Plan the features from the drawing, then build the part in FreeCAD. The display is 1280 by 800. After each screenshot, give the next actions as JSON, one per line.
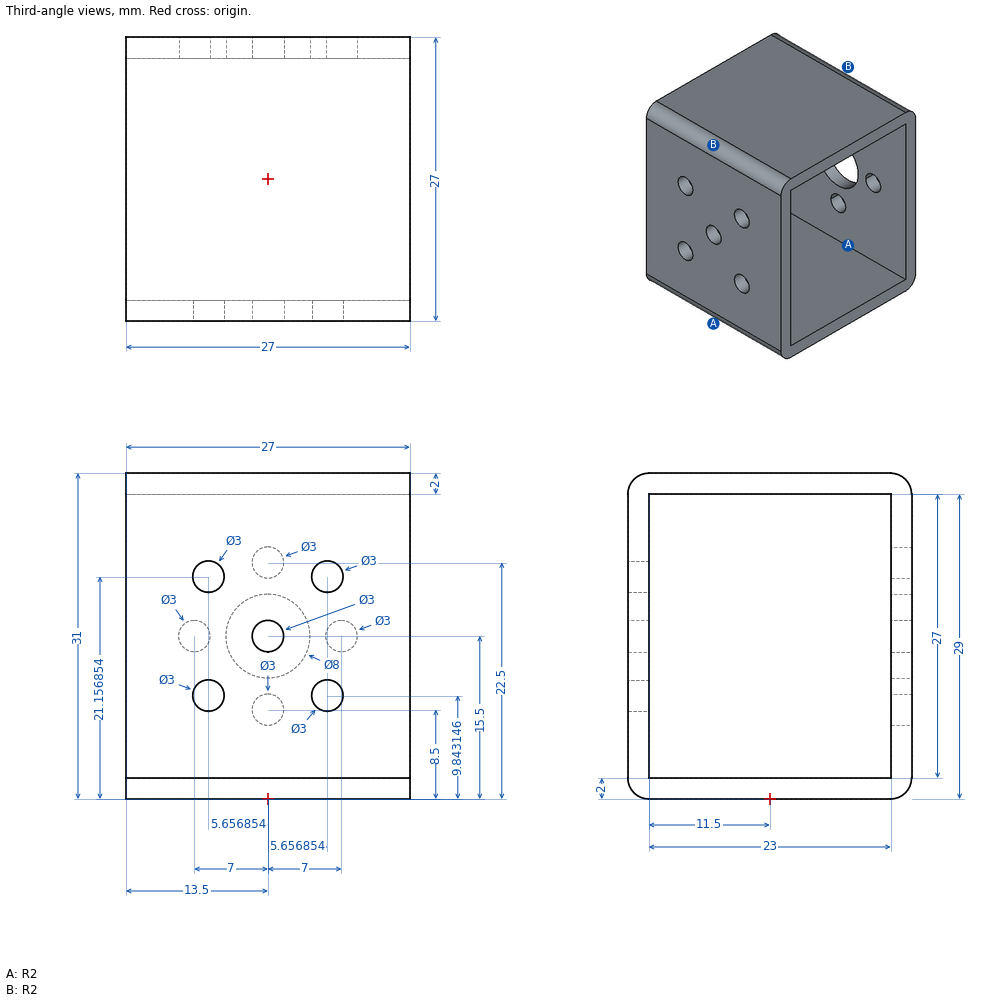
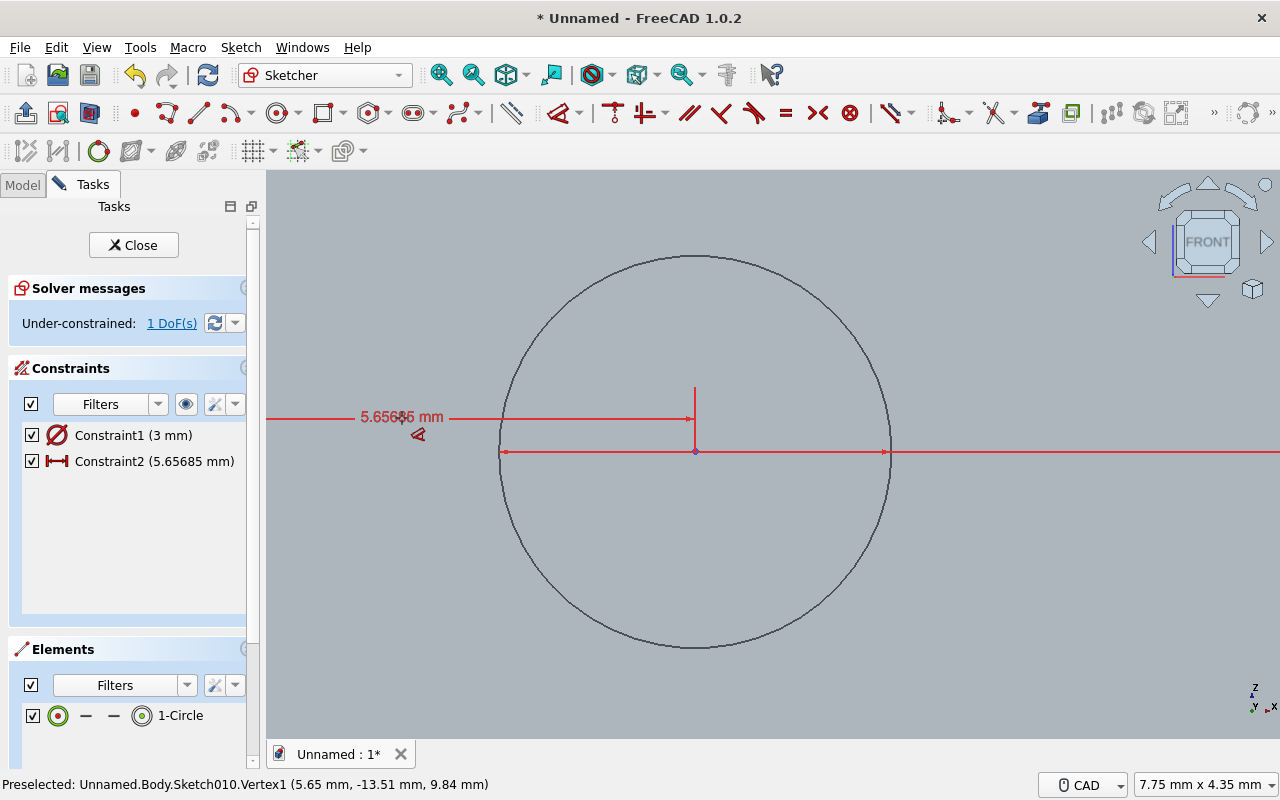
{"action": "left_click", "coordinate": [695, 452]}
{"action": "left_click", "coordinate": [729, 581]}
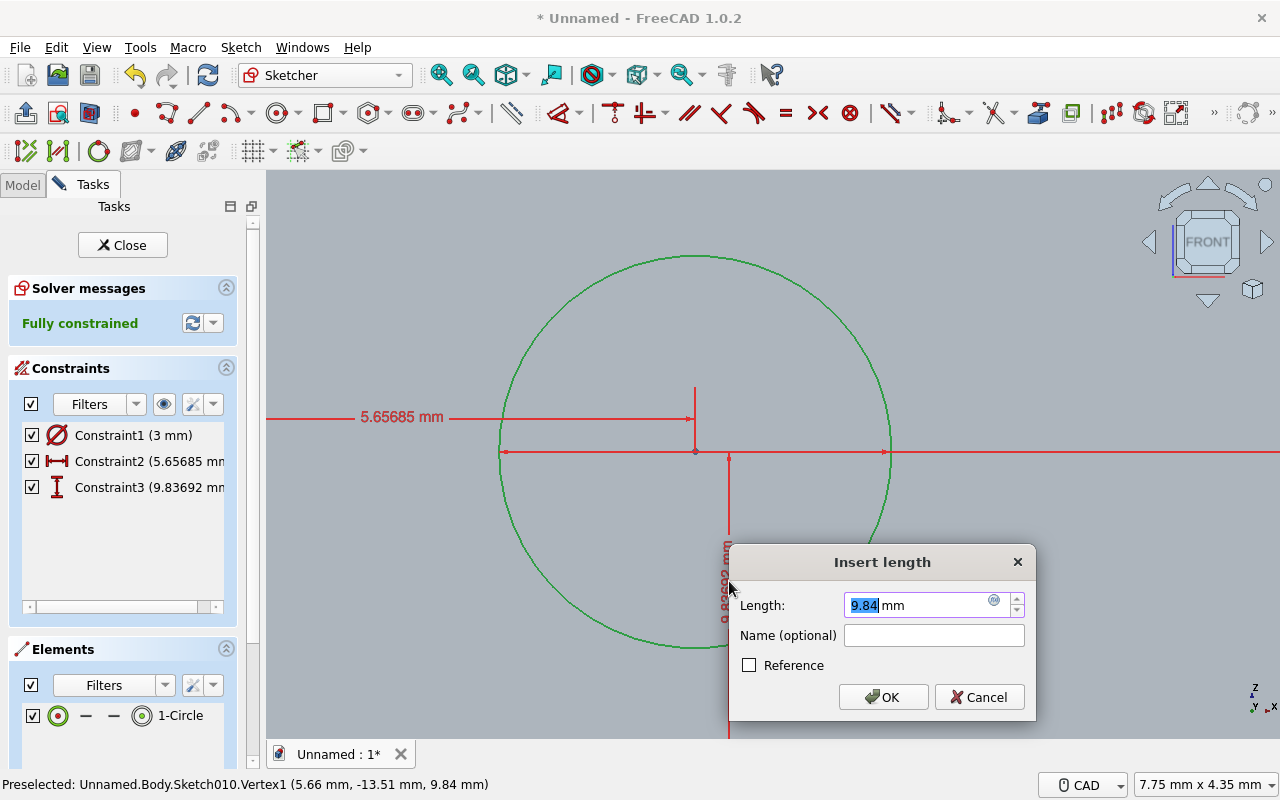
{"action": "type", "text": "9.843146"}
{"action": "key", "text": "Return"}
{"action": "key", "text": "Escape"}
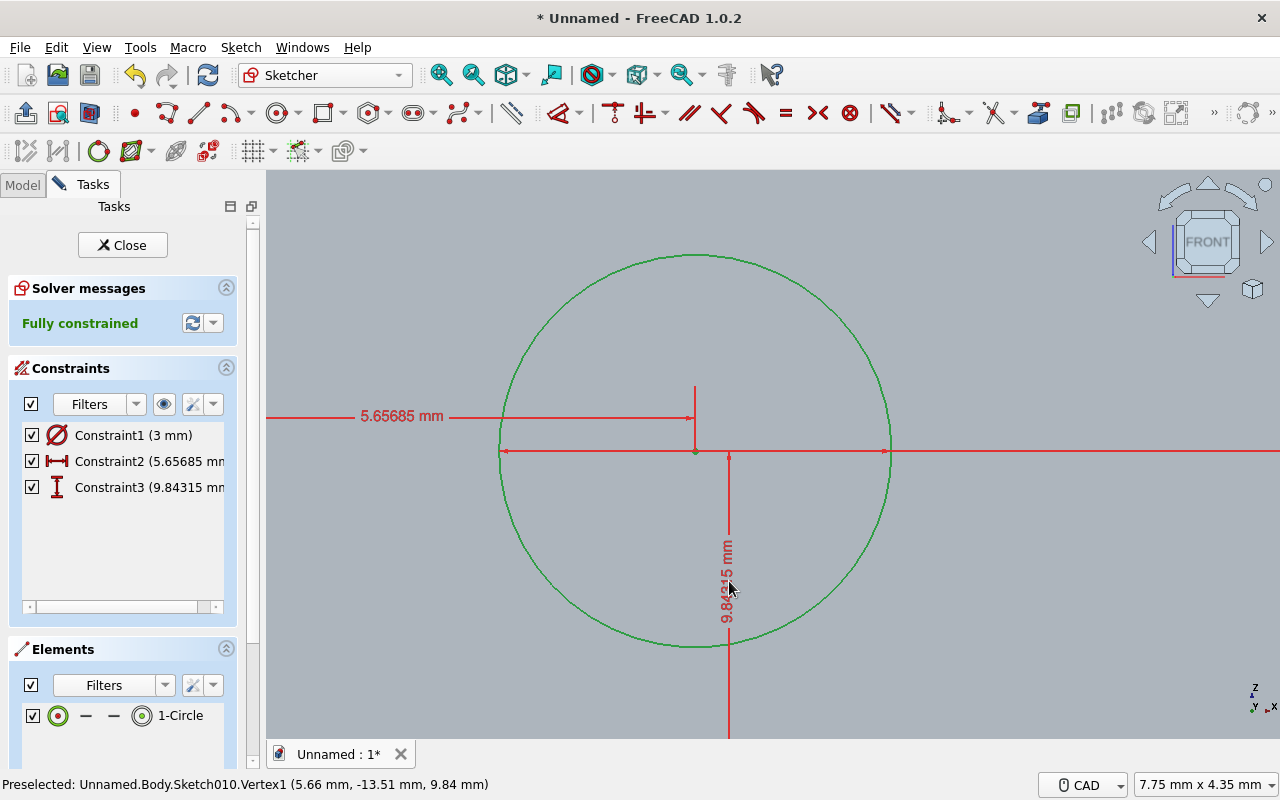
{"action": "left_click", "coordinate": [123, 245]}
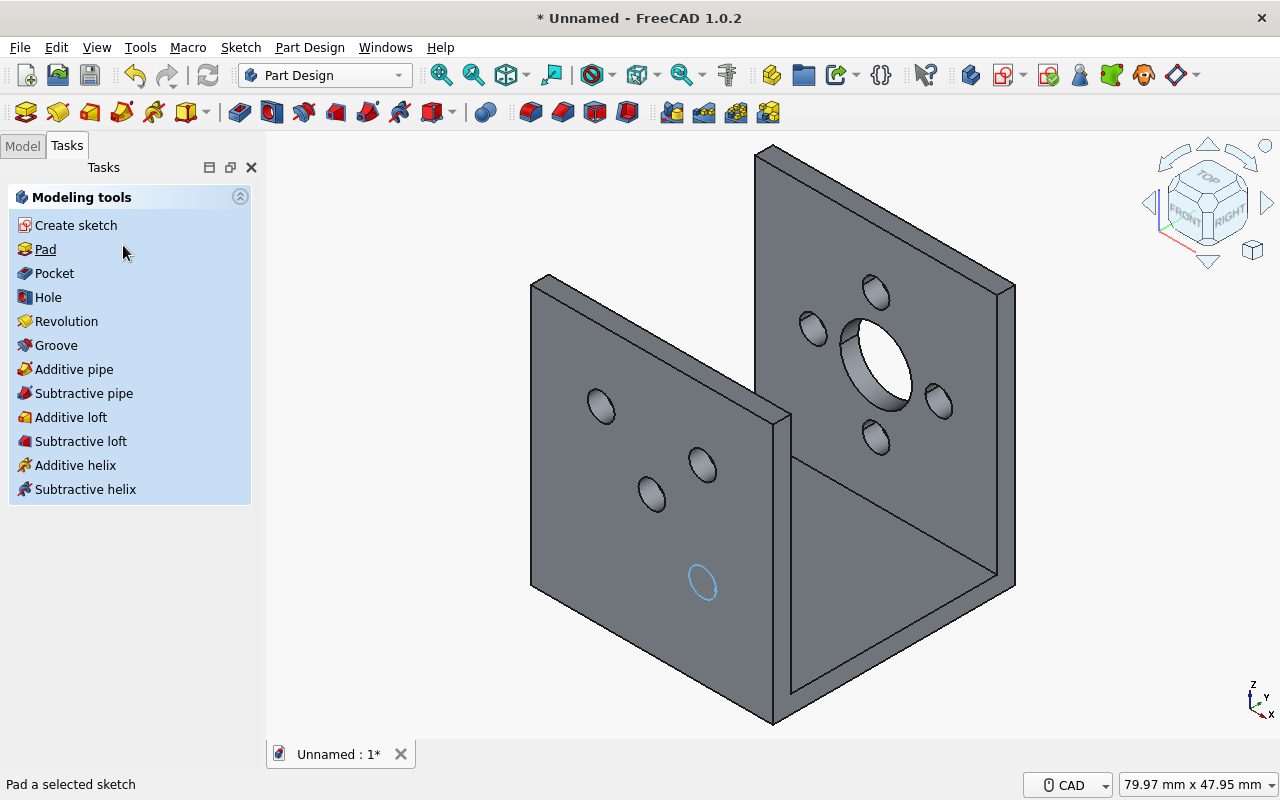
{"action": "left_click", "coordinate": [240, 112]}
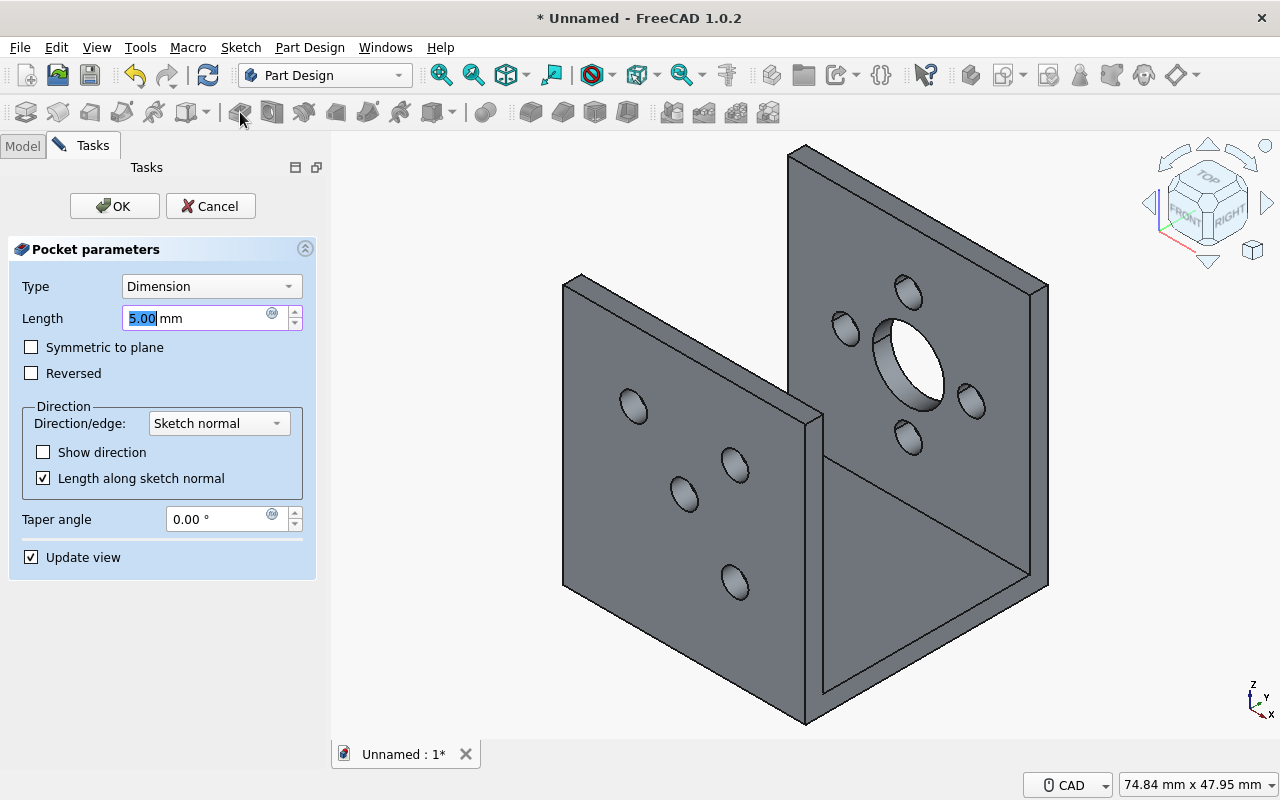
{"action": "left_click", "coordinate": [212, 286]}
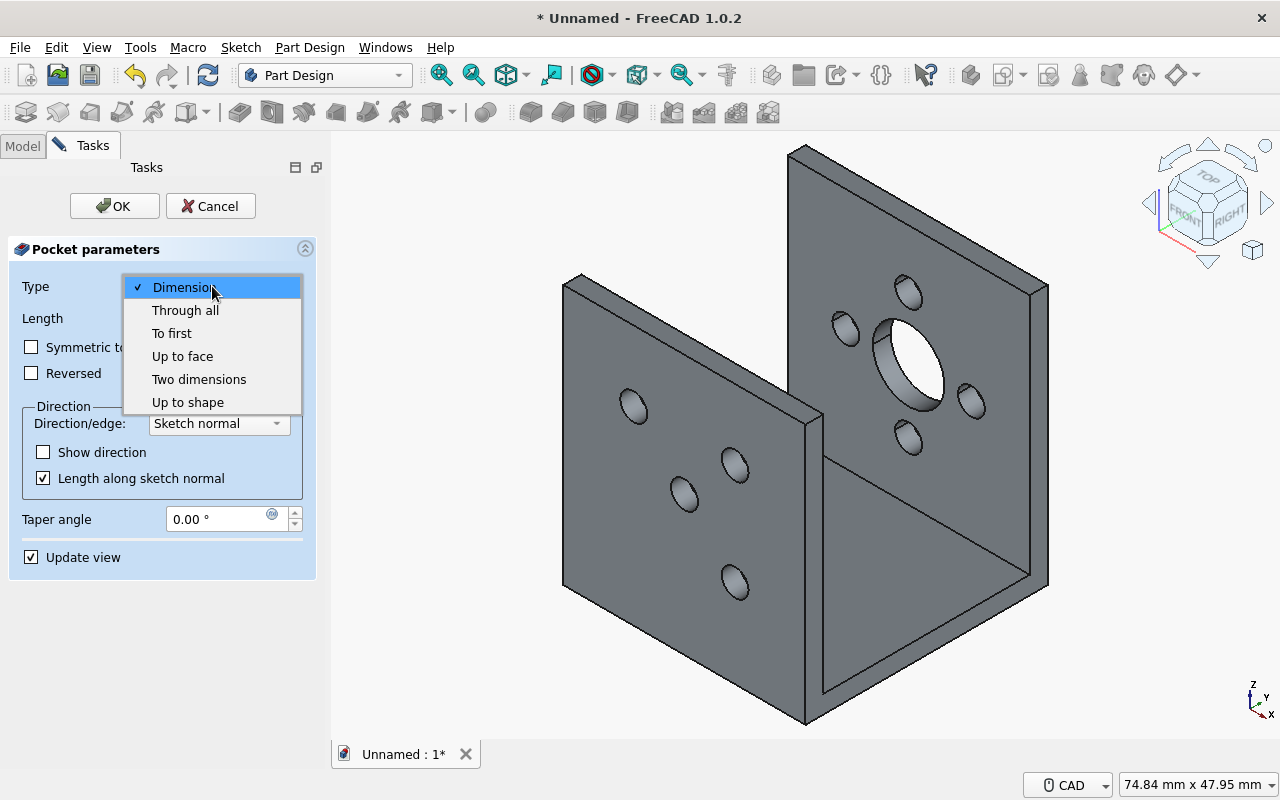
{"action": "left_click", "coordinate": [212, 334]}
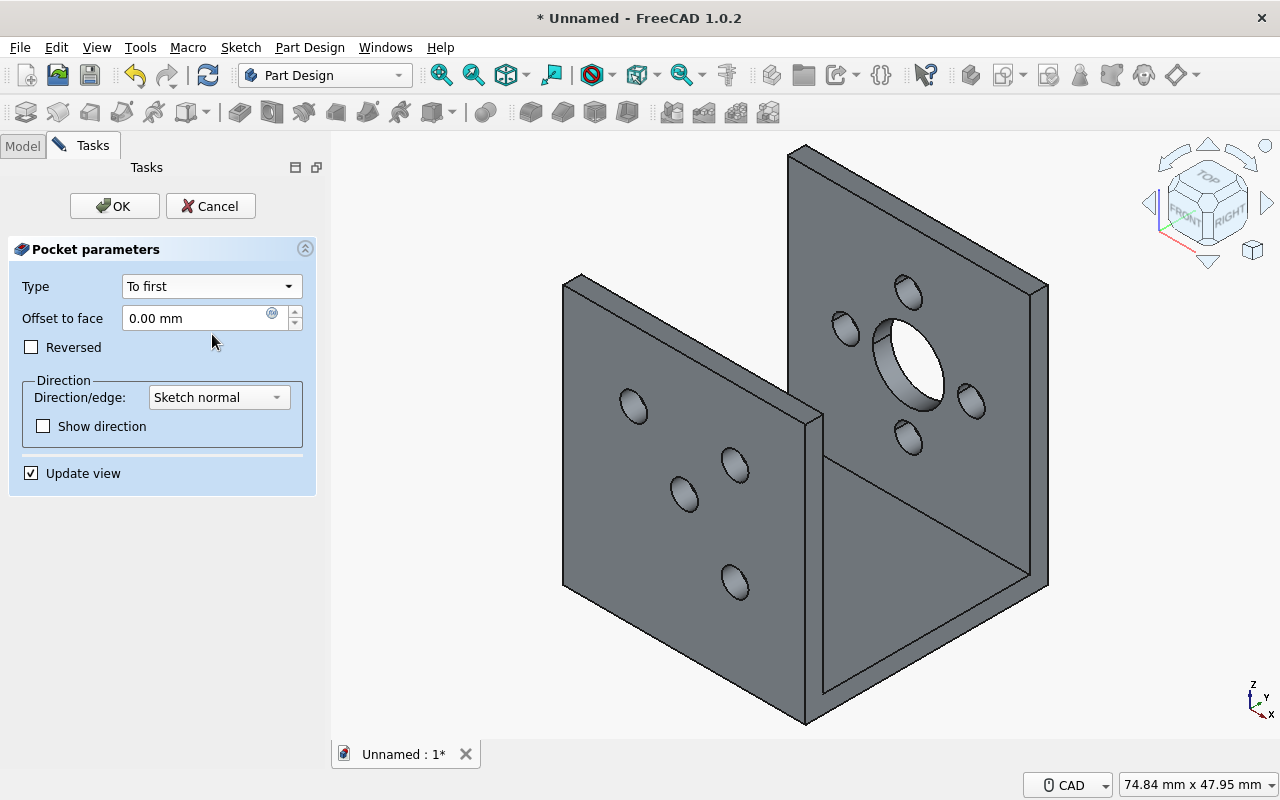
{"action": "left_click", "coordinate": [115, 206]}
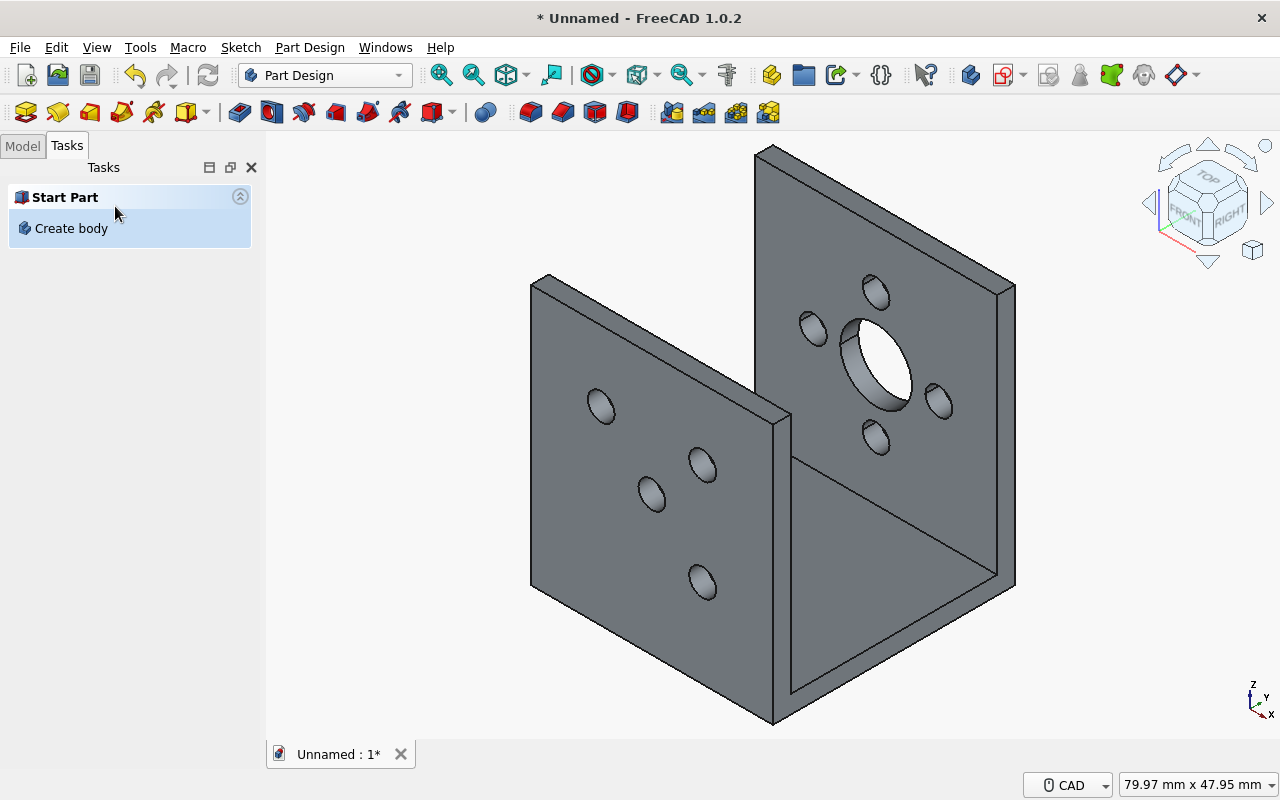
{"action": "left_click", "coordinate": [617, 570]}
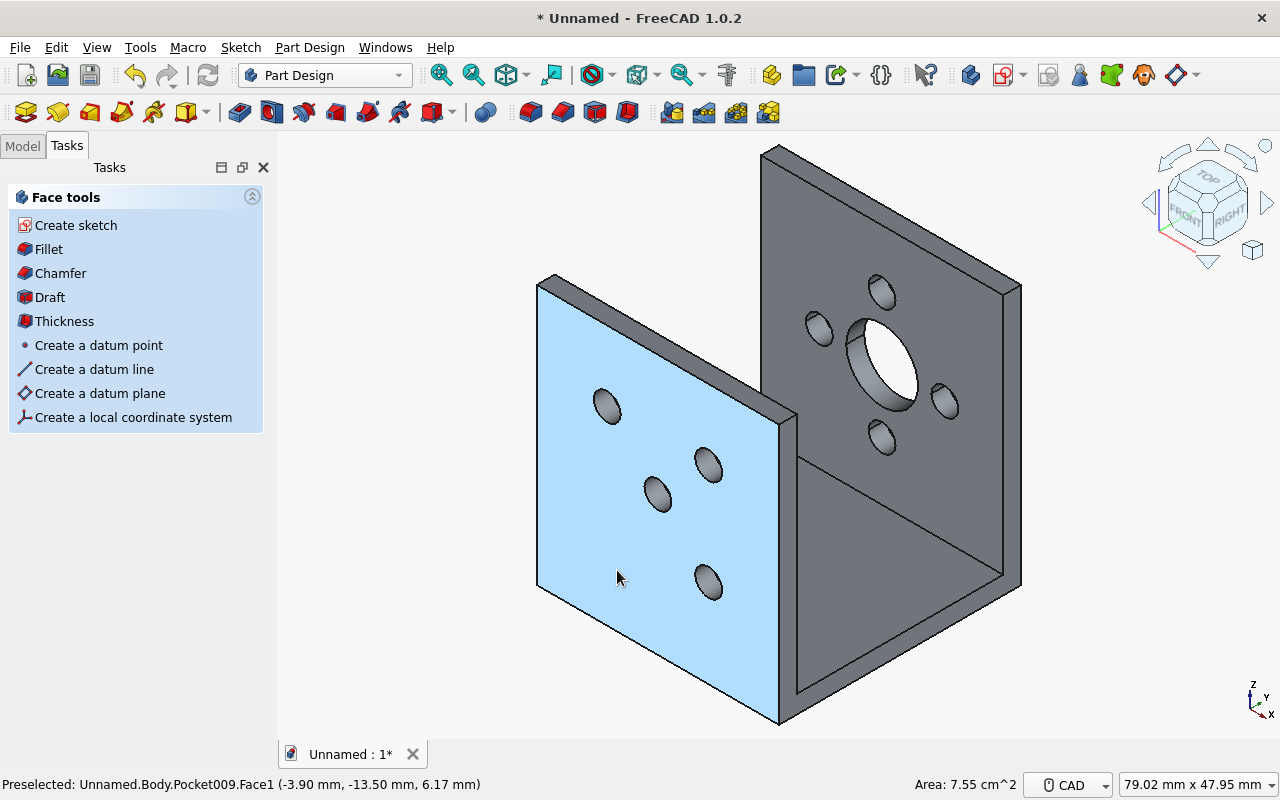
{"action": "left_click", "coordinate": [1004, 76]}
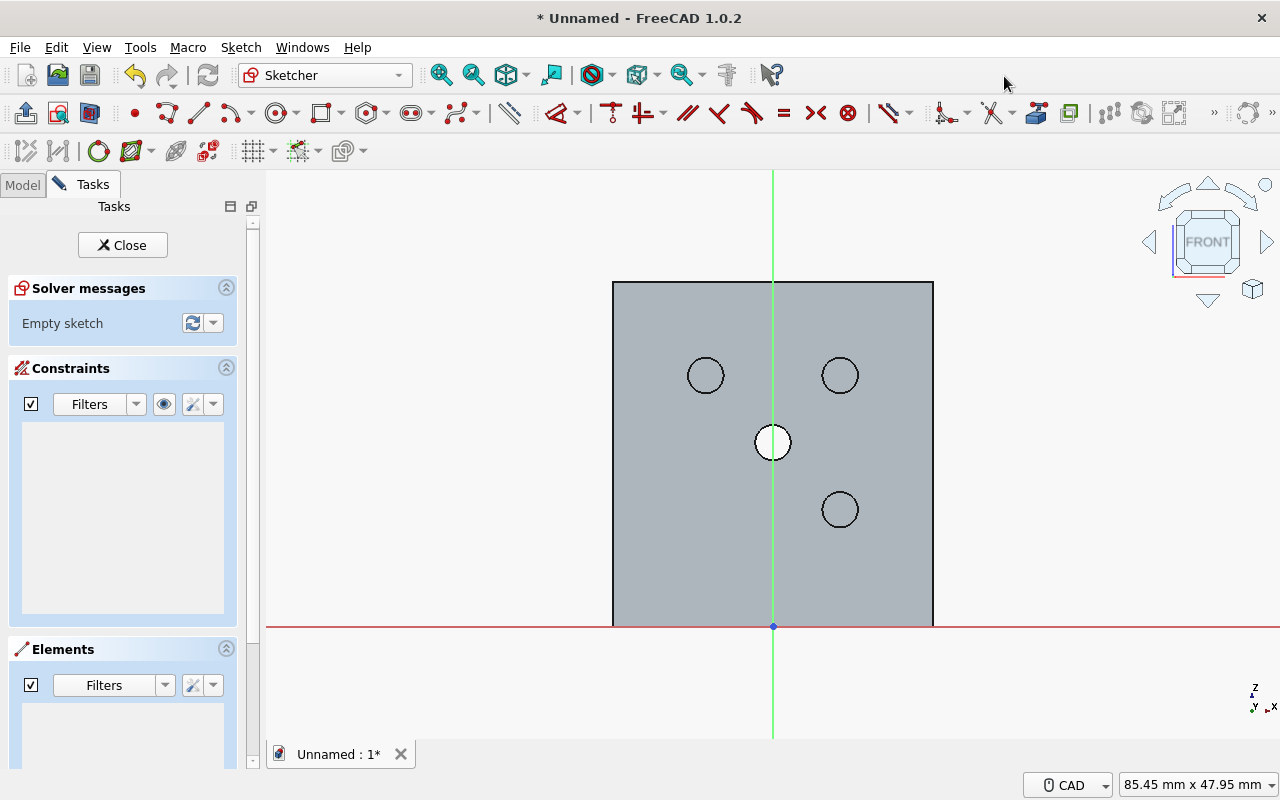
{"action": "scroll", "coordinate": [706, 515], "scroll_direction": "up", "scroll_amount": 12}